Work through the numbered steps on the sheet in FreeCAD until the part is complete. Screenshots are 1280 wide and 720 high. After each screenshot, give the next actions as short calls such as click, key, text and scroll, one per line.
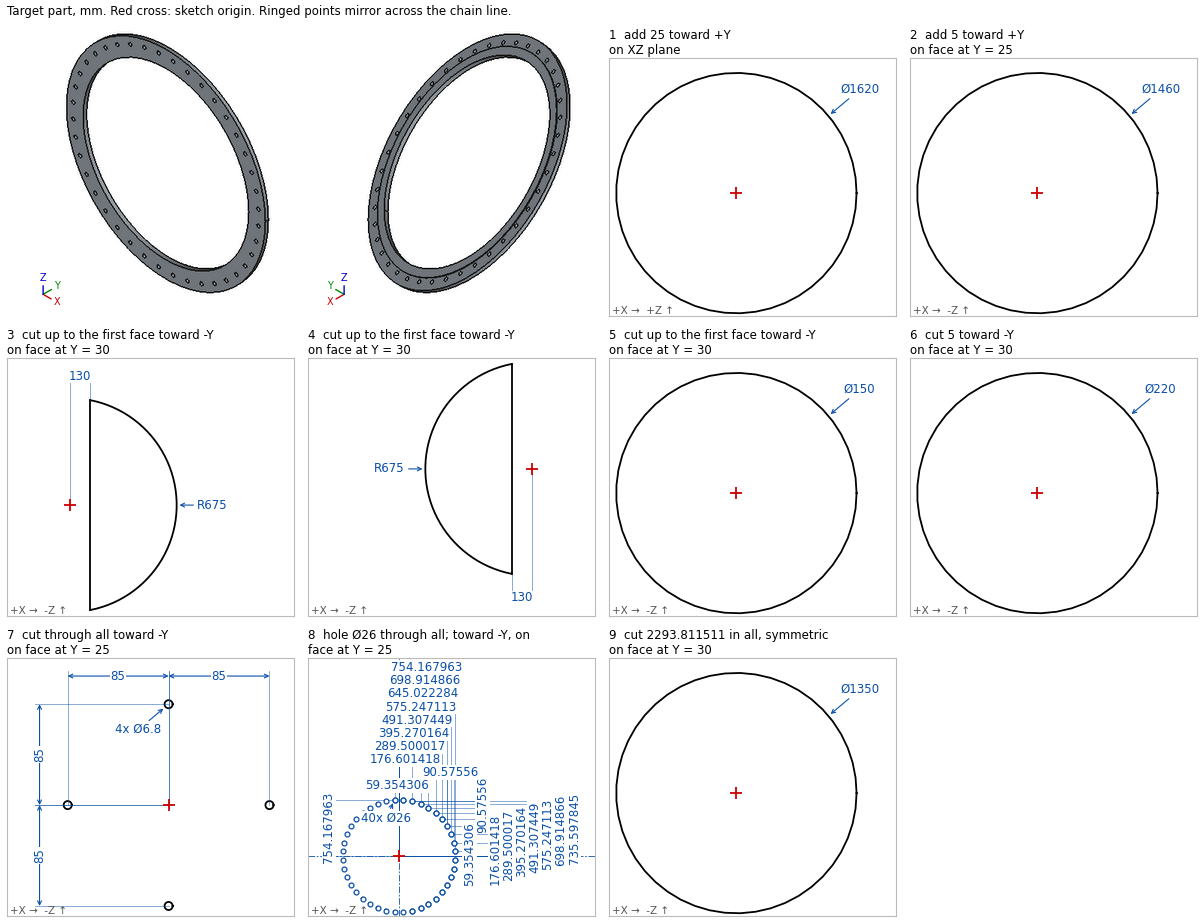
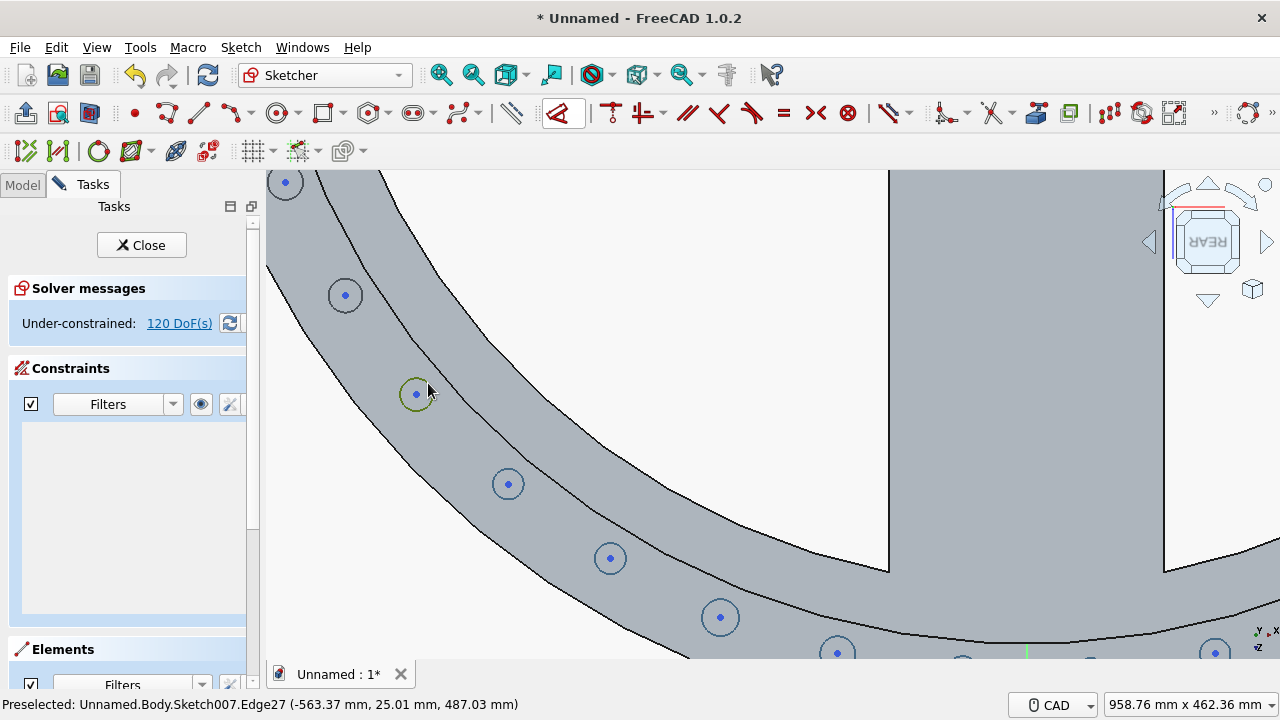
click(357, 284)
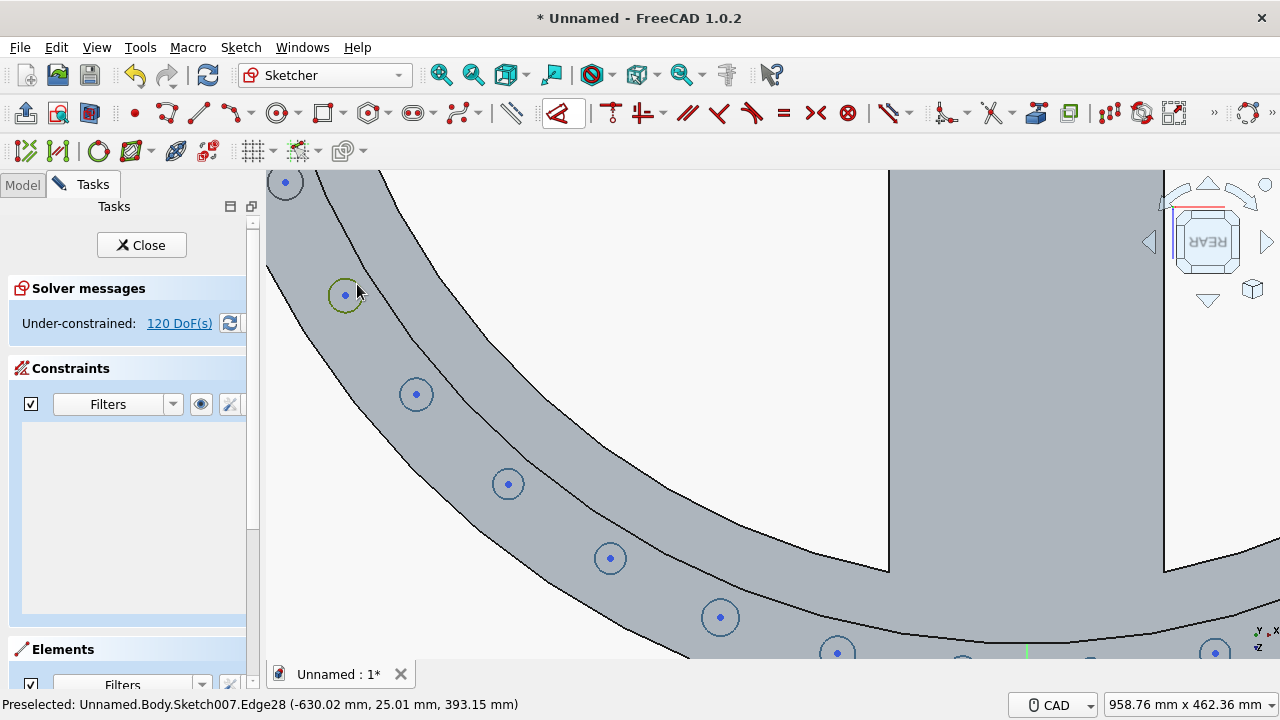
scroll(623, 552, down, 8)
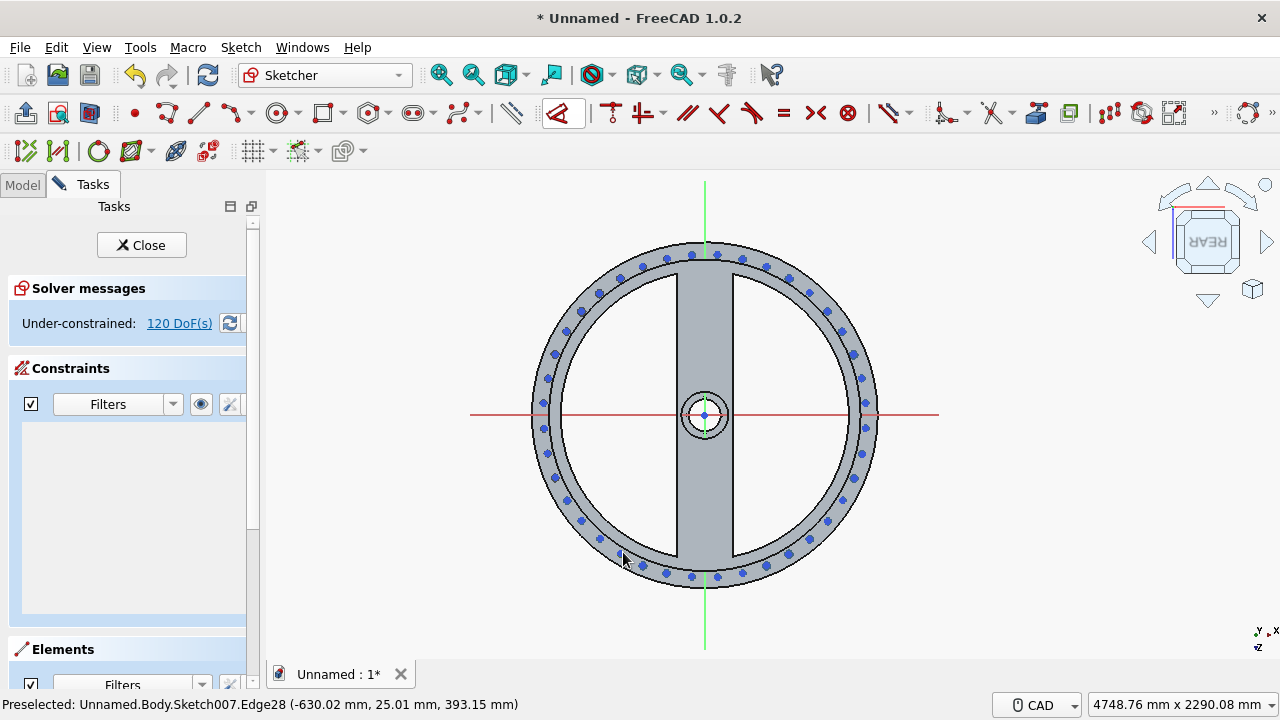
scroll(558, 475, up, 7)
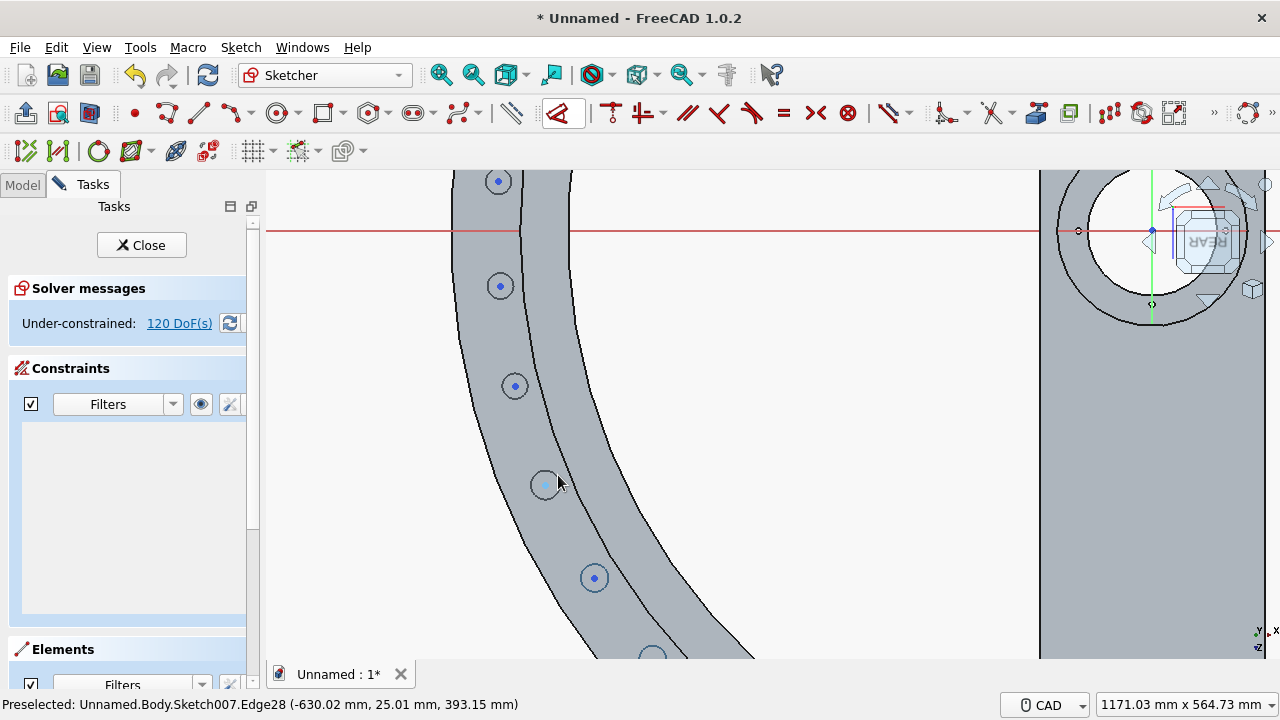
click(556, 475)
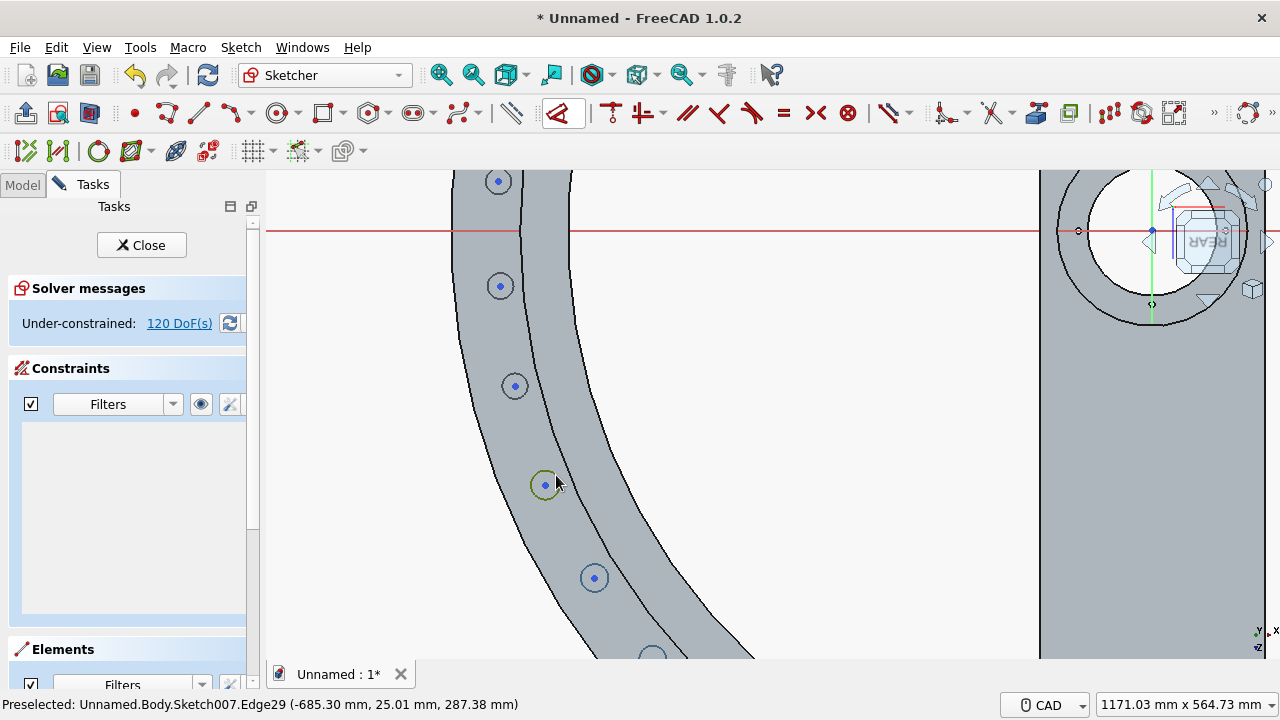
click(524, 377)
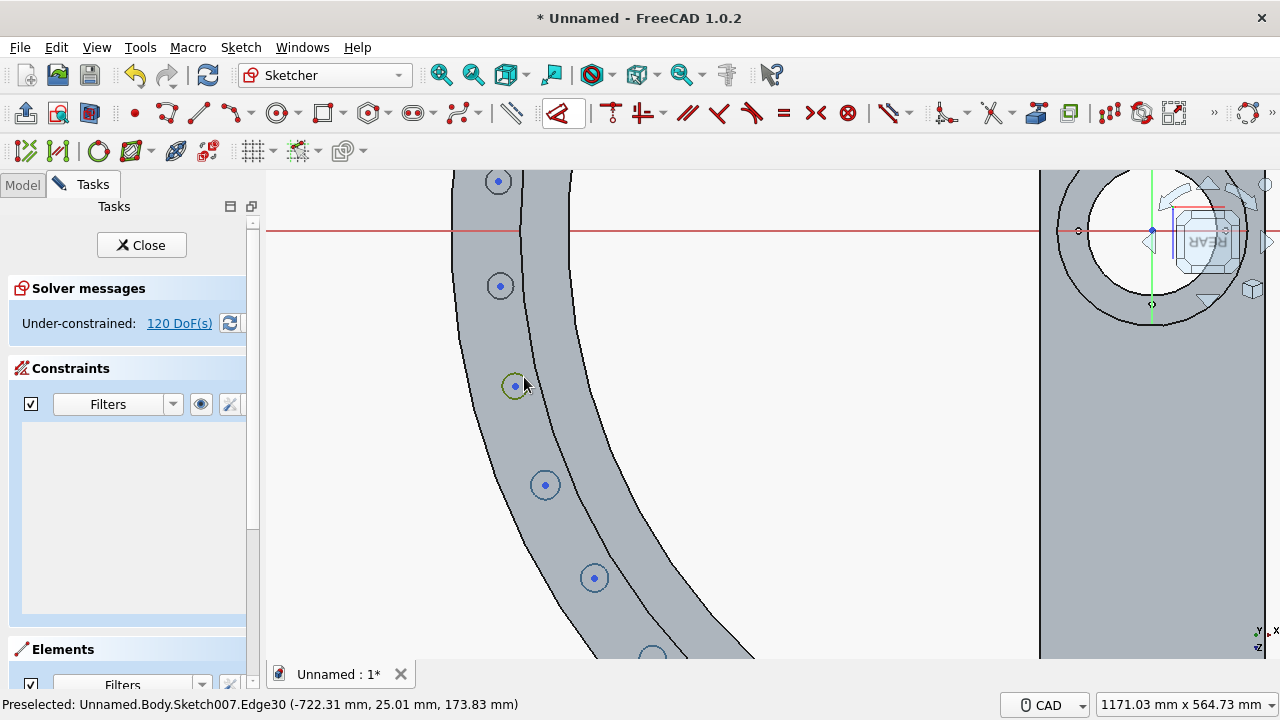
click(510, 277)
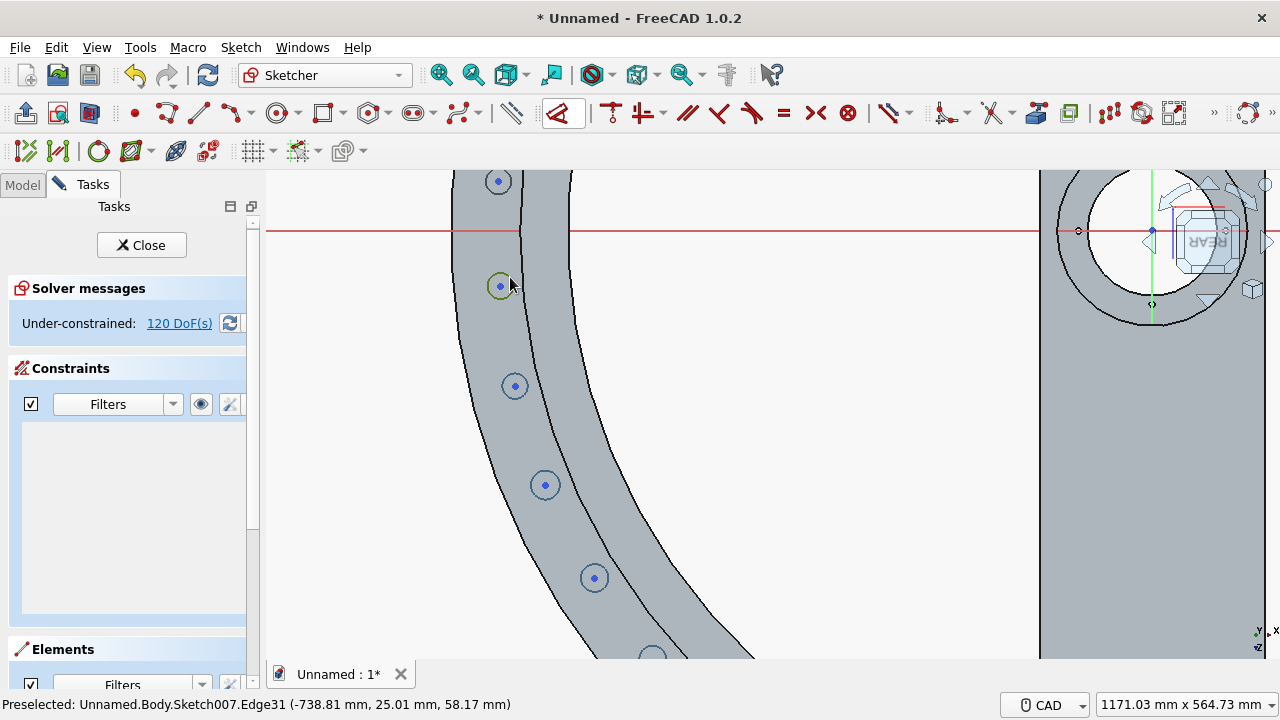
scroll(558, 475, down, 7)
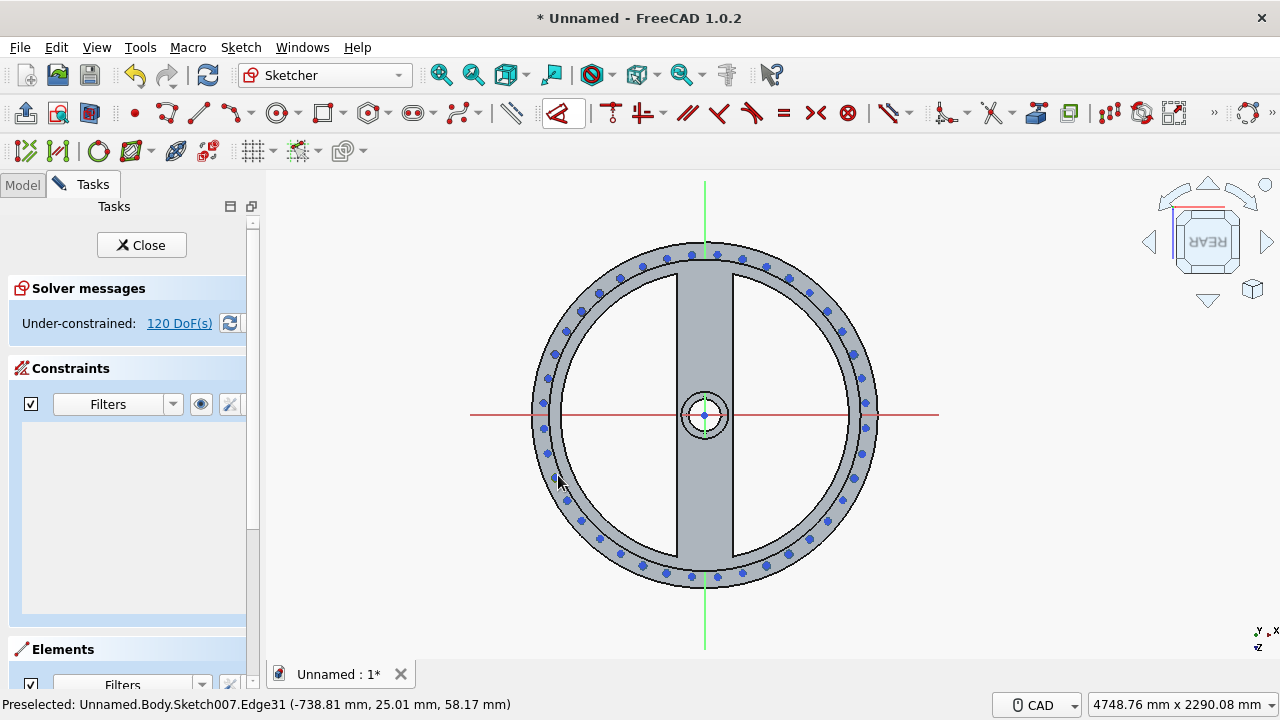
scroll(546, 401, up, 8)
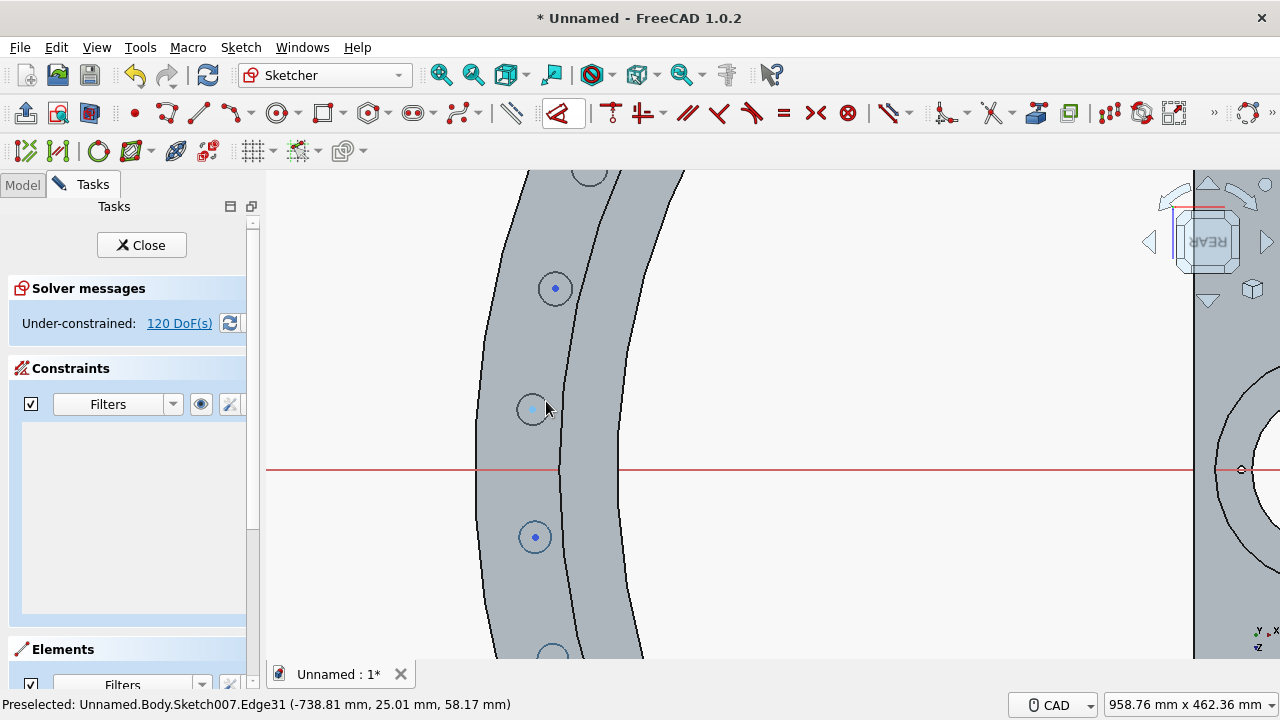
click(544, 399)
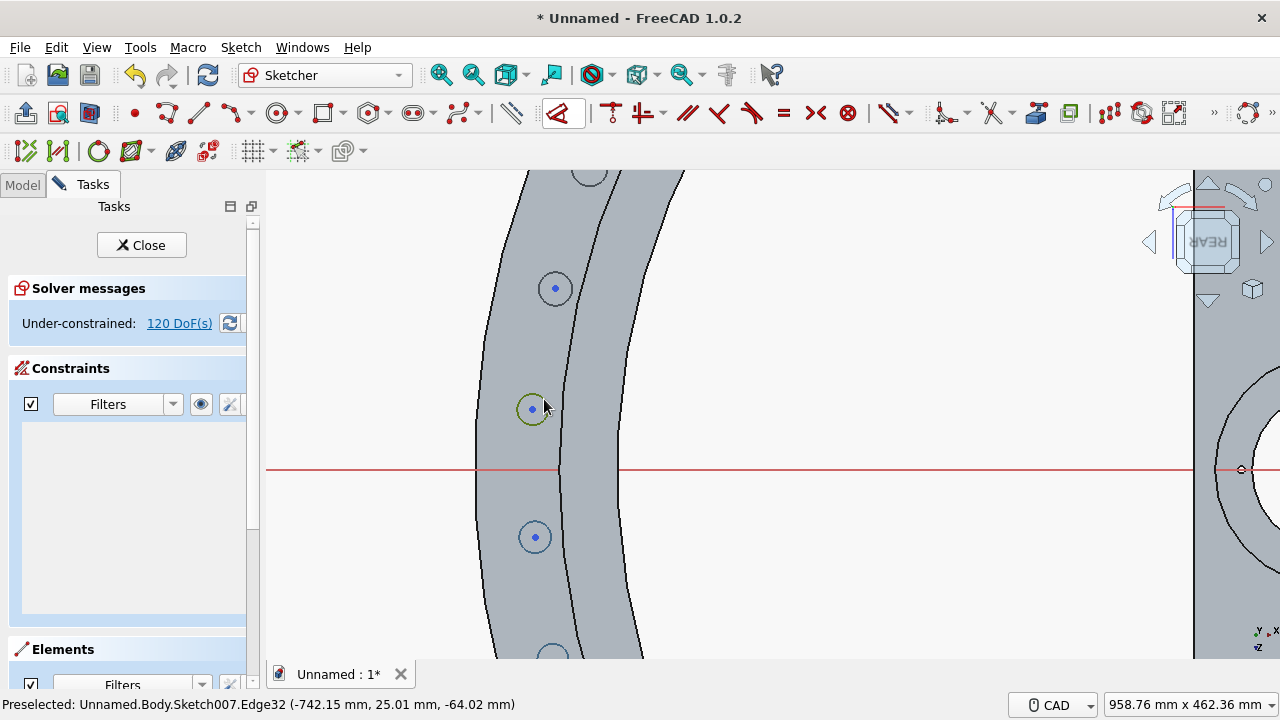
click(567, 277)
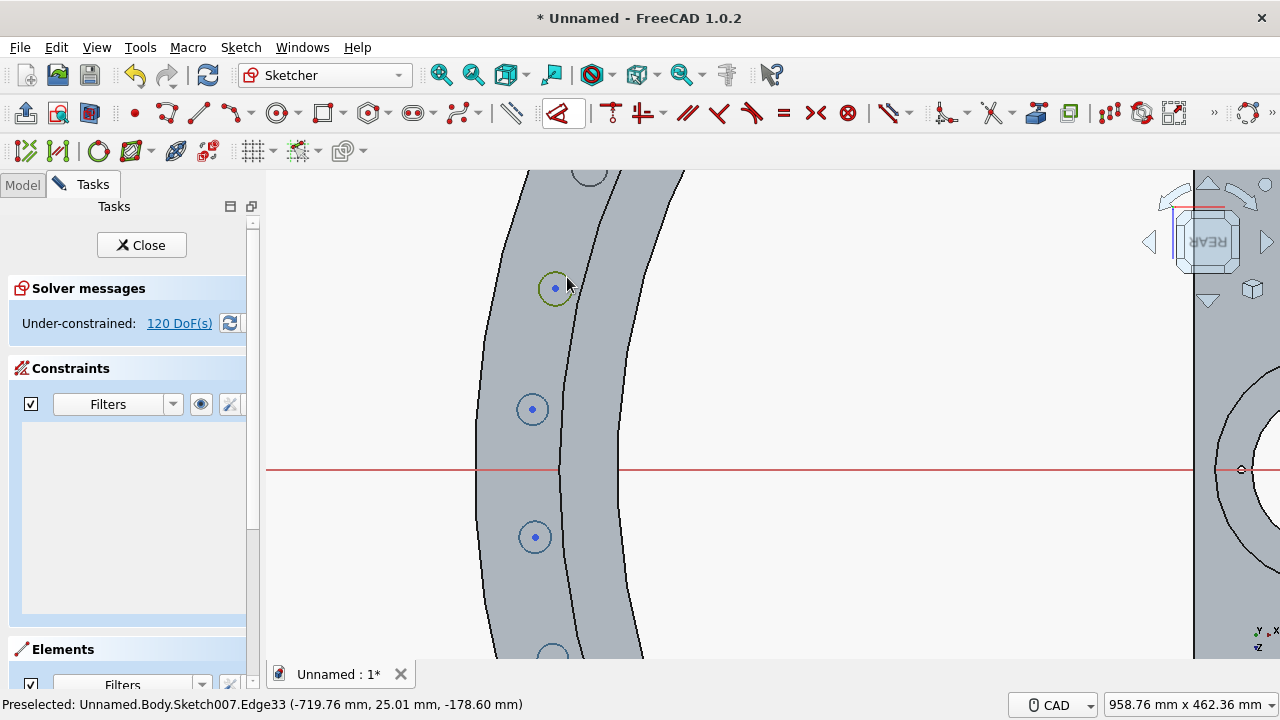
scroll(546, 400, down, 8)